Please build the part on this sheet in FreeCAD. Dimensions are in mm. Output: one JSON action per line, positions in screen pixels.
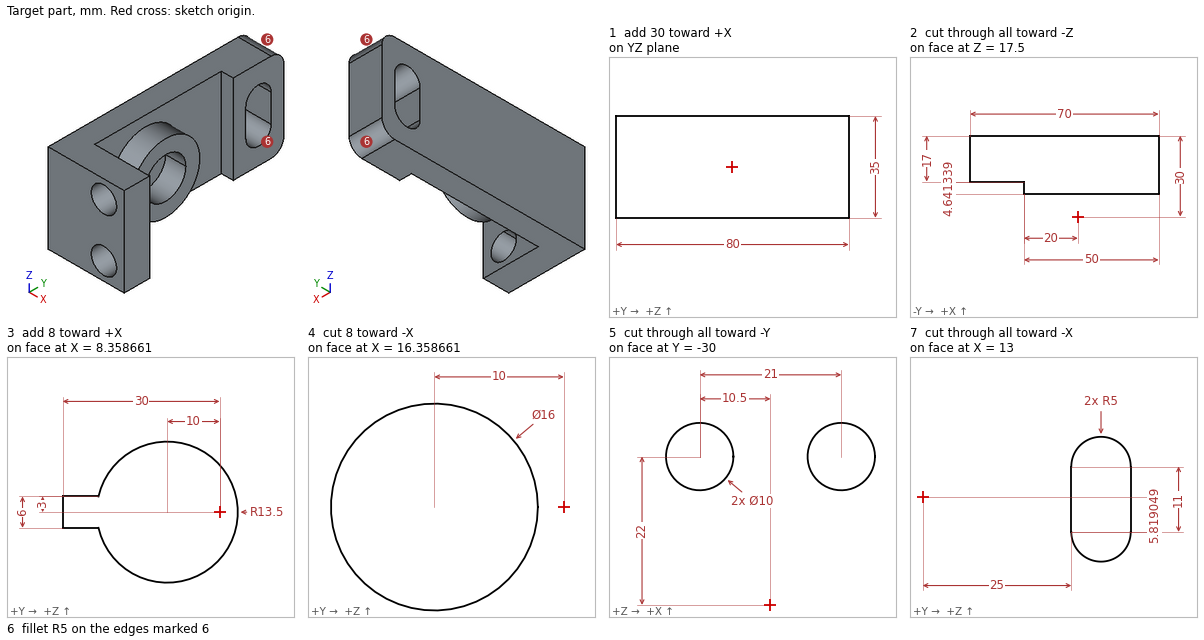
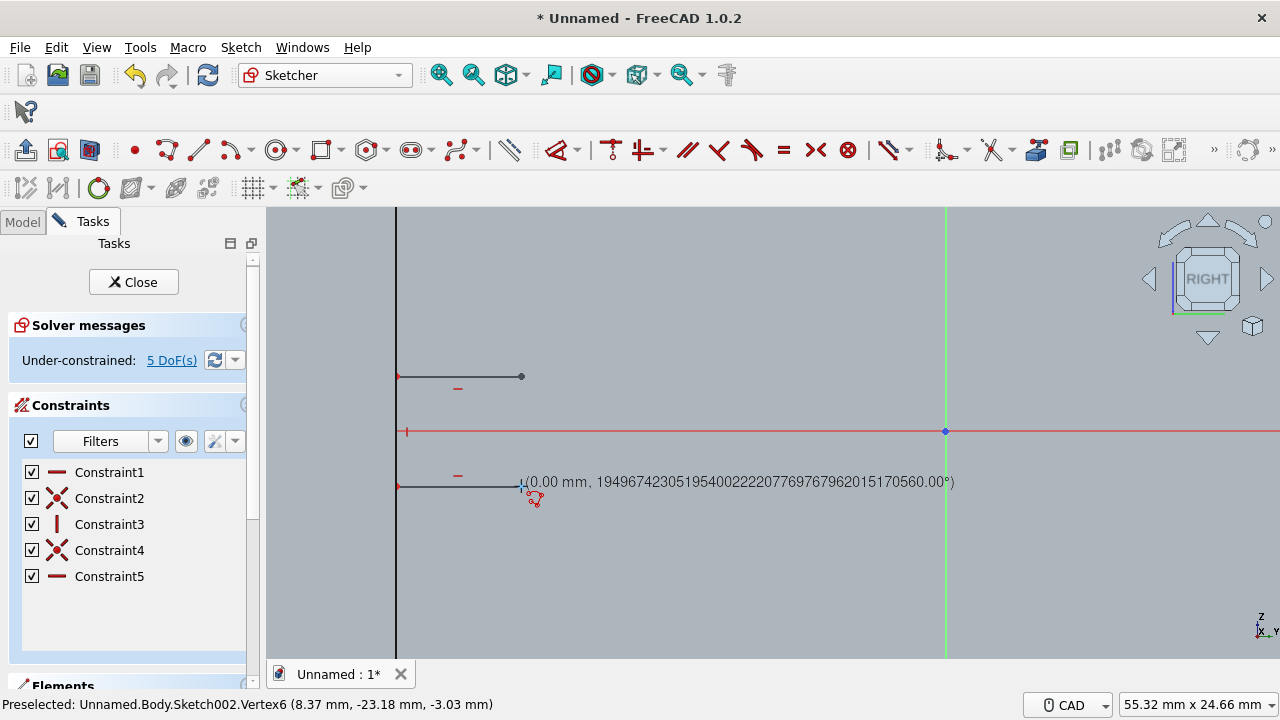
{"action": "left_click", "coordinate": [254, 150]}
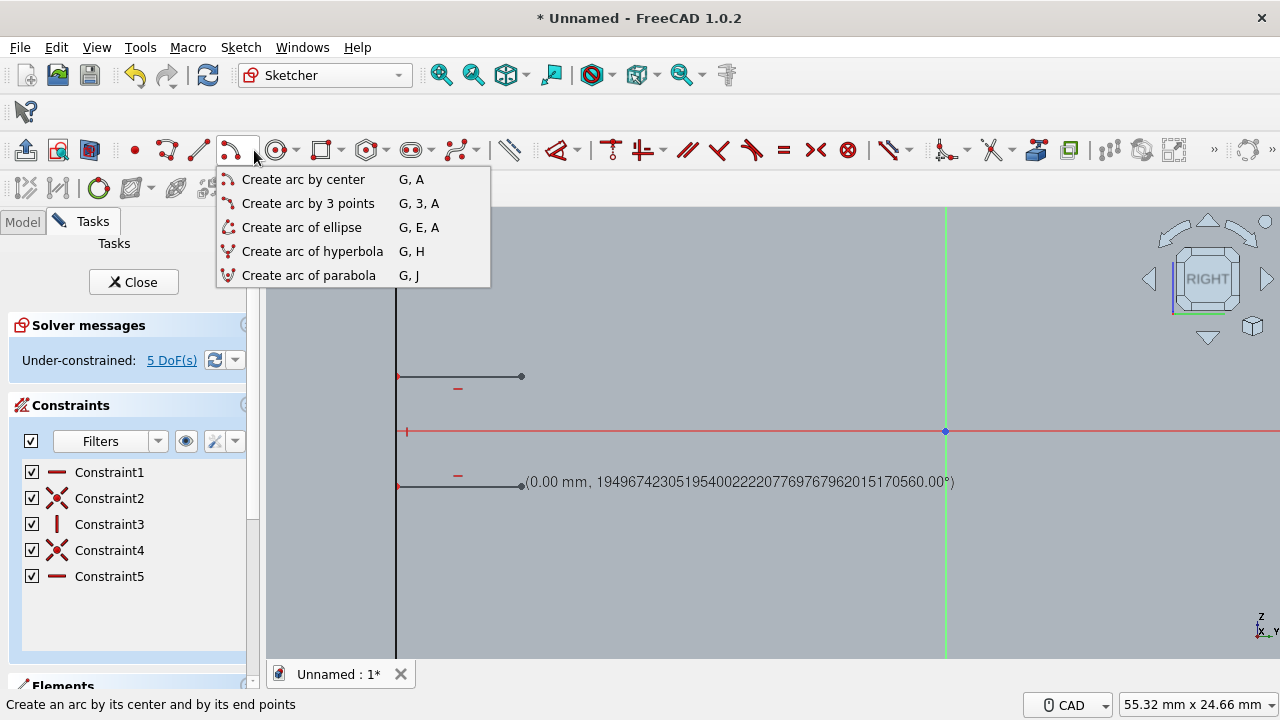
{"action": "left_click", "coordinate": [354, 203]}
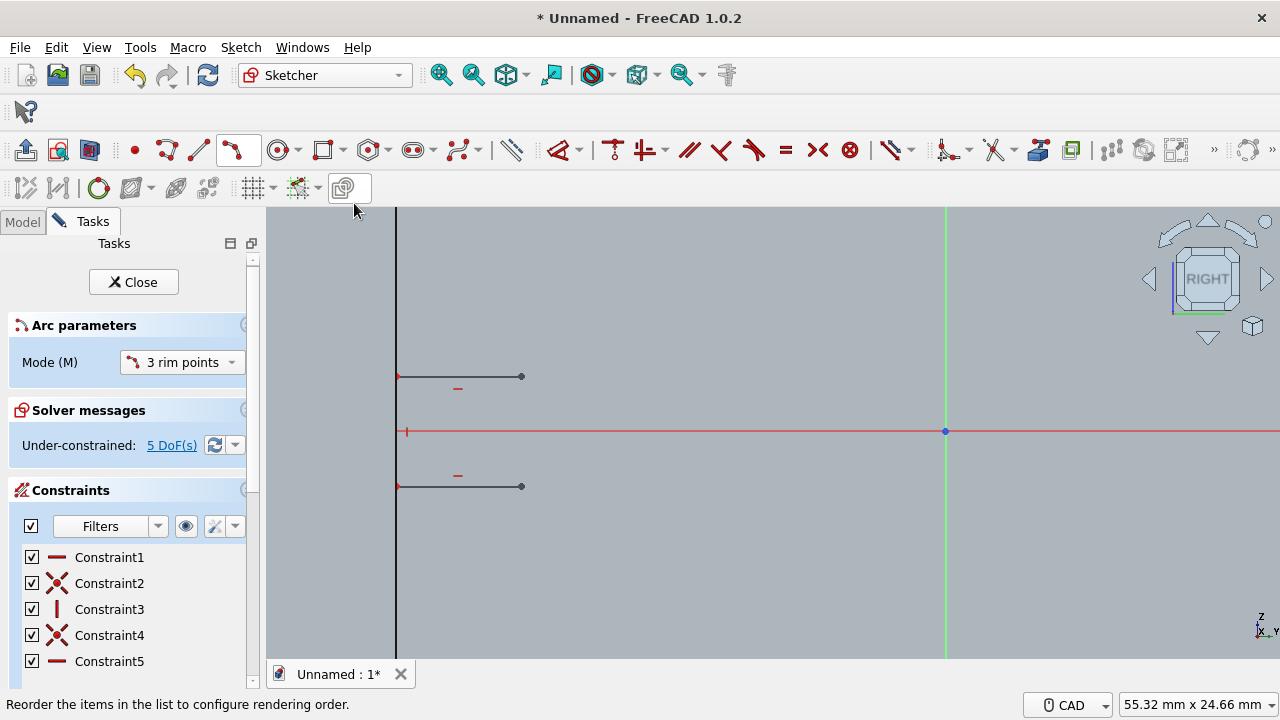
{"action": "left_click", "coordinate": [521, 487]}
{"action": "left_click", "coordinate": [521, 377]}
{"action": "left_click", "coordinate": [969, 568]}
{"action": "key", "text": "Escape"}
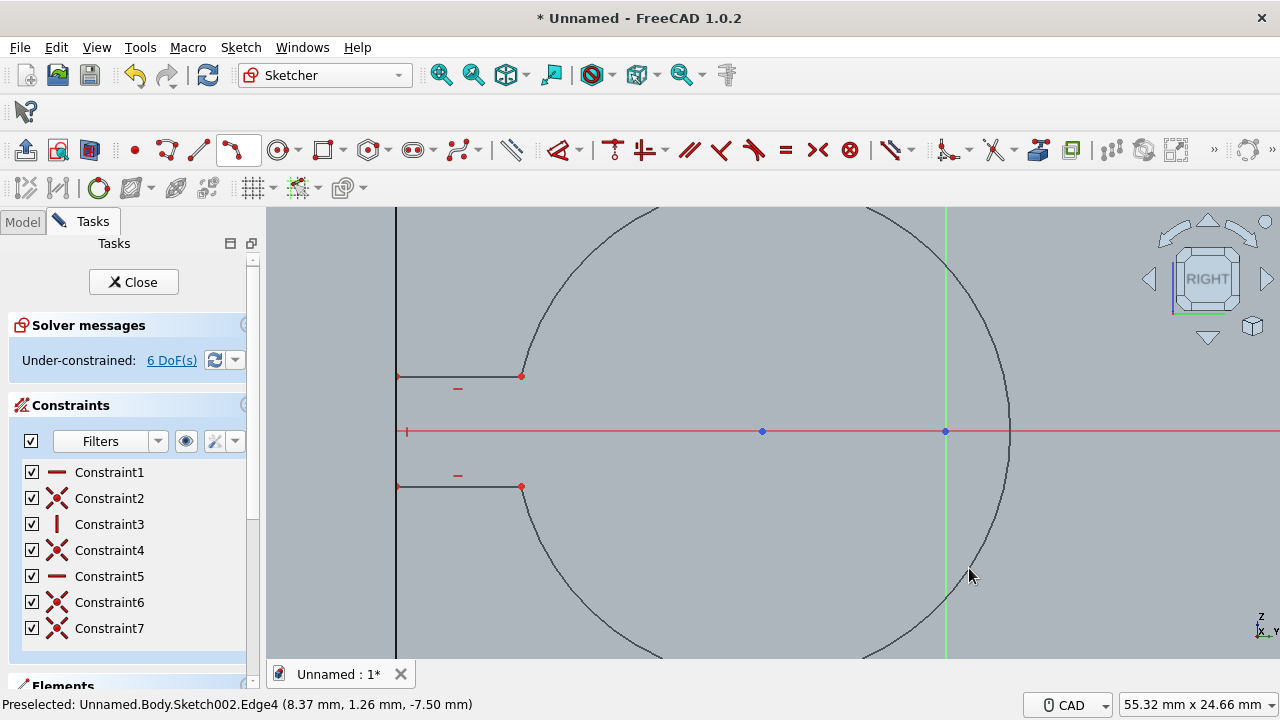
{"action": "left_click", "coordinate": [763, 432]}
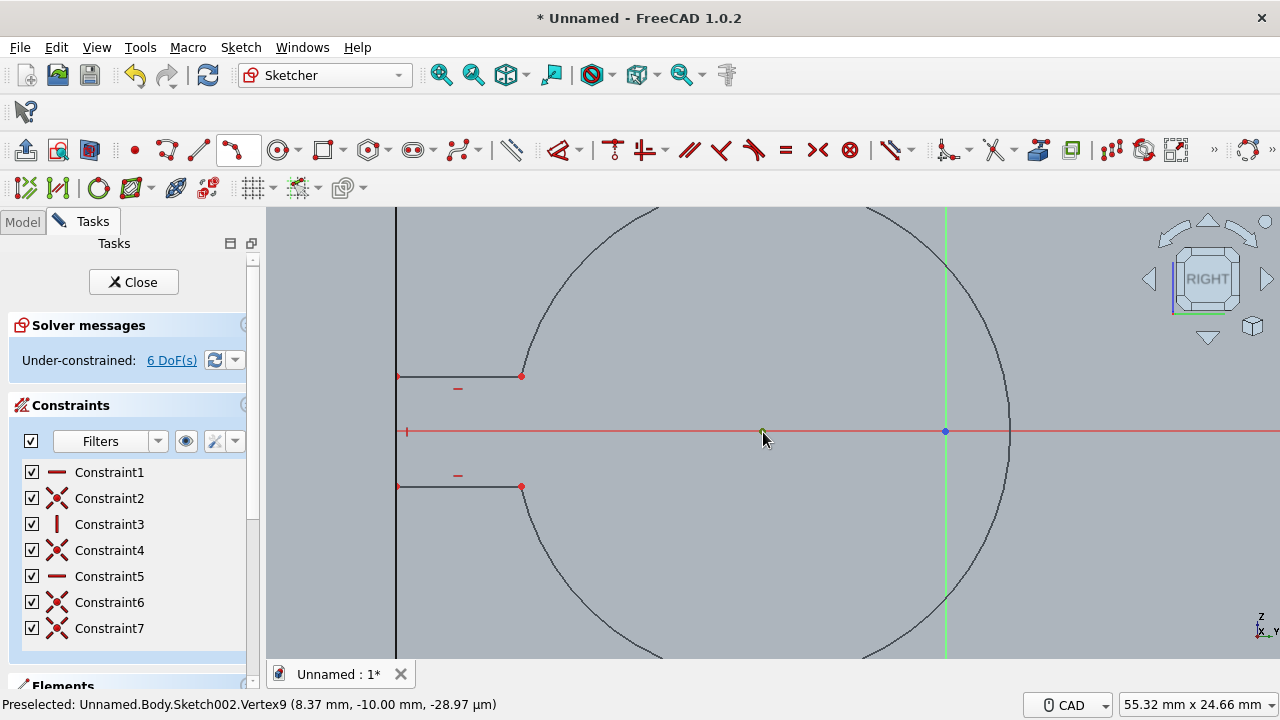
{"action": "left_click", "coordinate": [353, 431]}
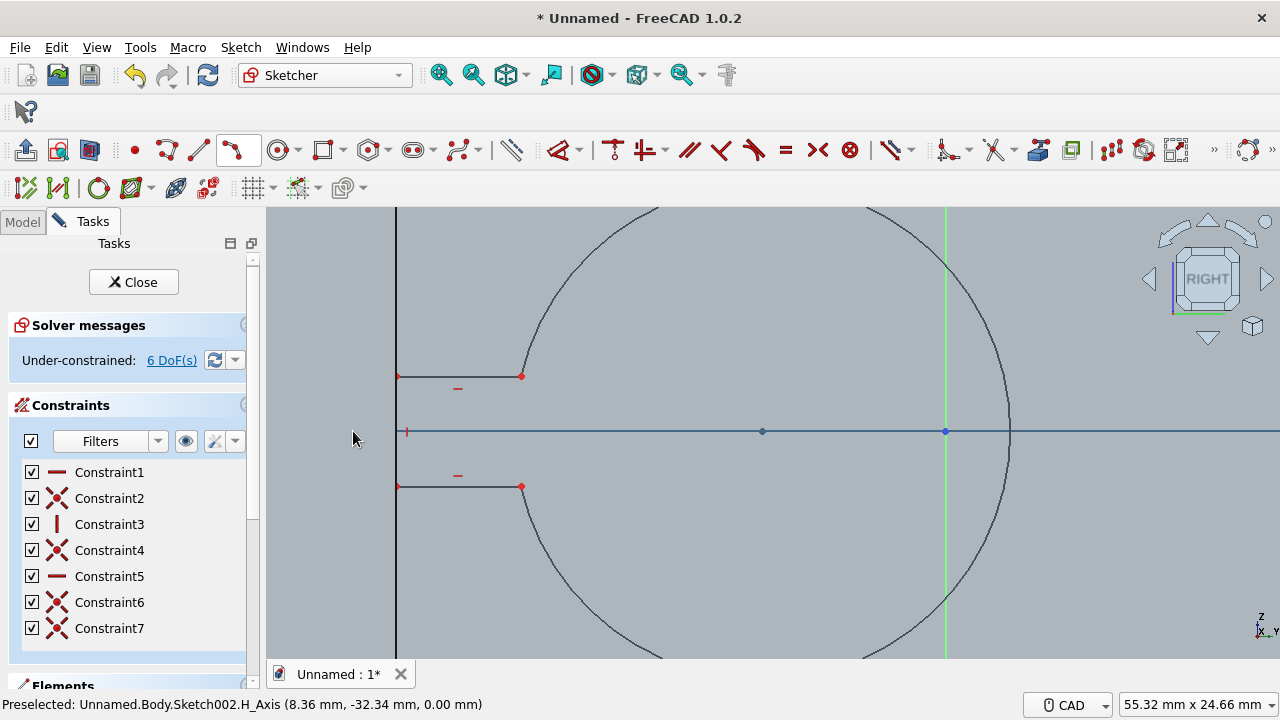
{"action": "left_click", "coordinate": [614, 150]}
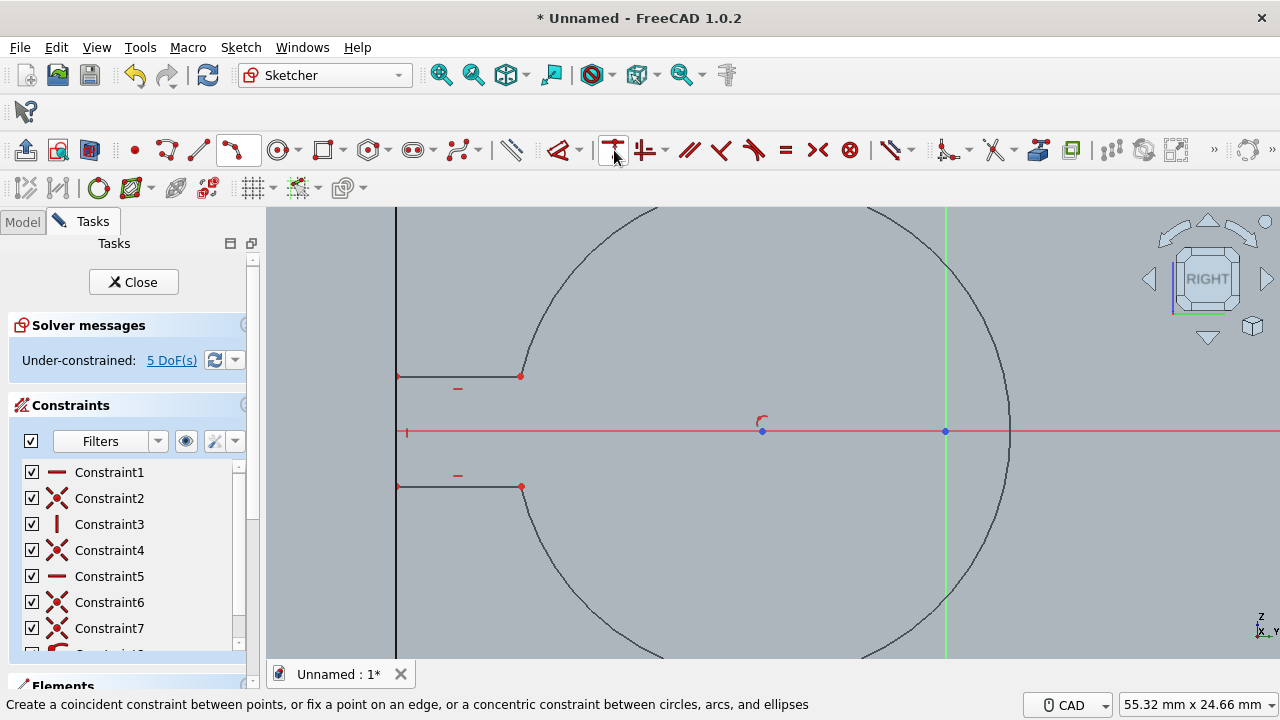
{"action": "left_click", "coordinate": [558, 150]}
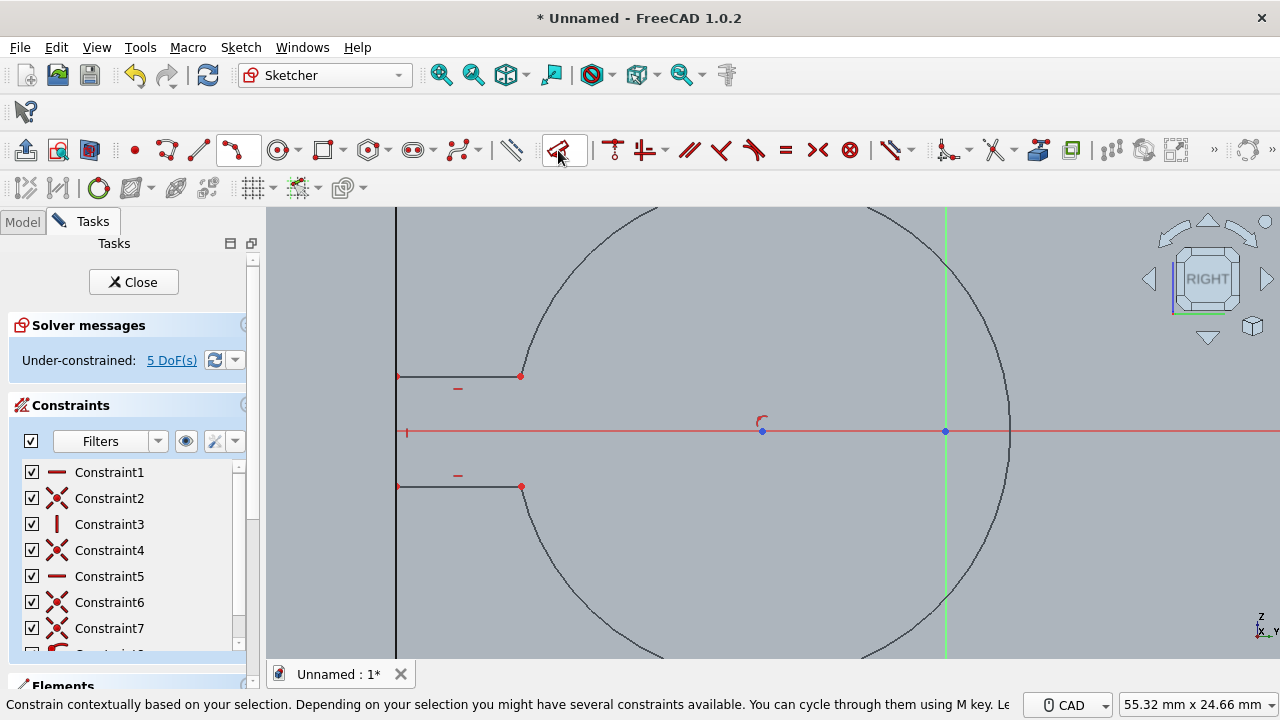
{"action": "left_click", "coordinate": [1010, 431]}
{"action": "left_click", "coordinate": [1008, 565]}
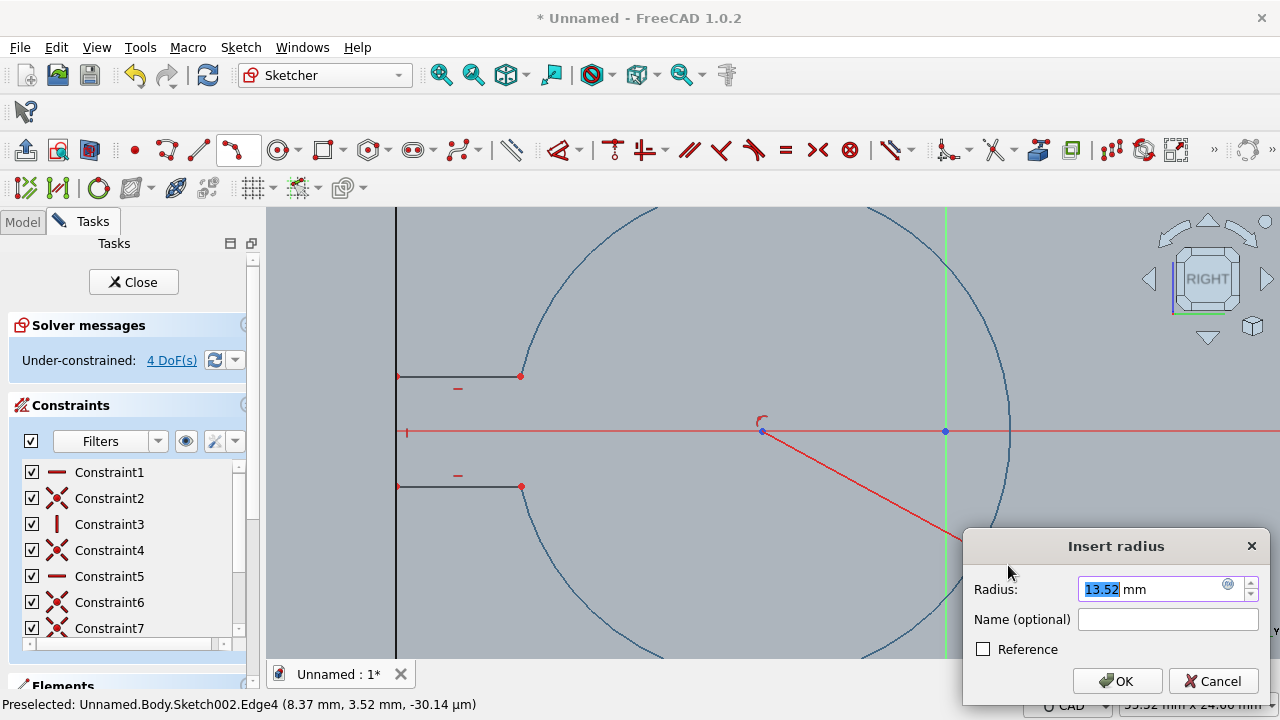
{"action": "type", "text": "13.5"}
{"action": "key", "text": "Return"}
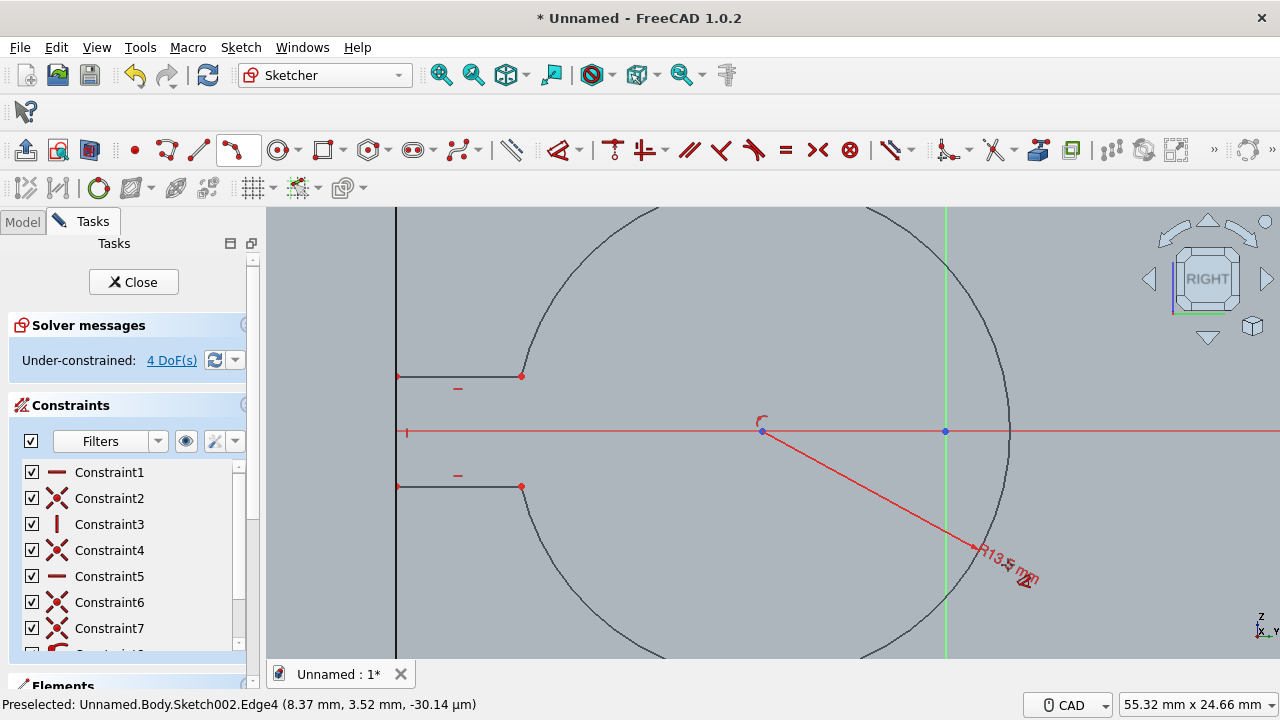
{"action": "left_click", "coordinate": [396, 410]}
{"action": "left_click", "coordinate": [362, 407]}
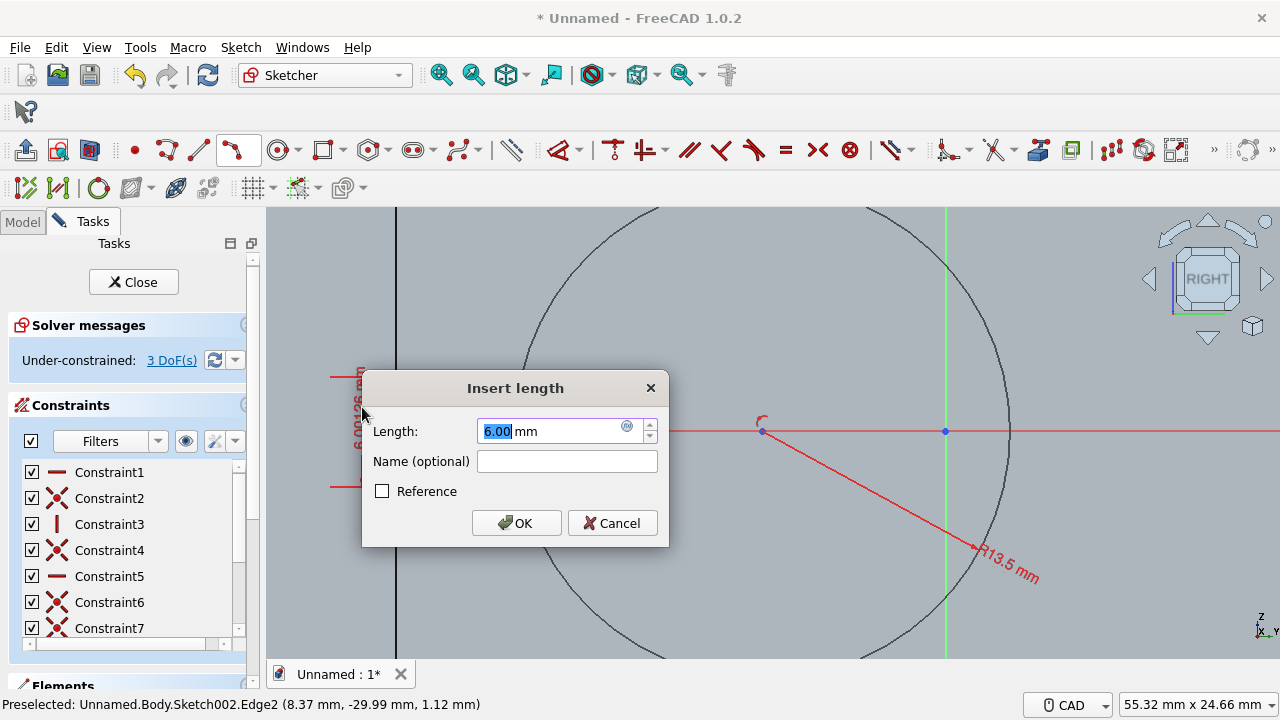
{"action": "type", "text": "6"}
{"action": "key", "text": "Return"}